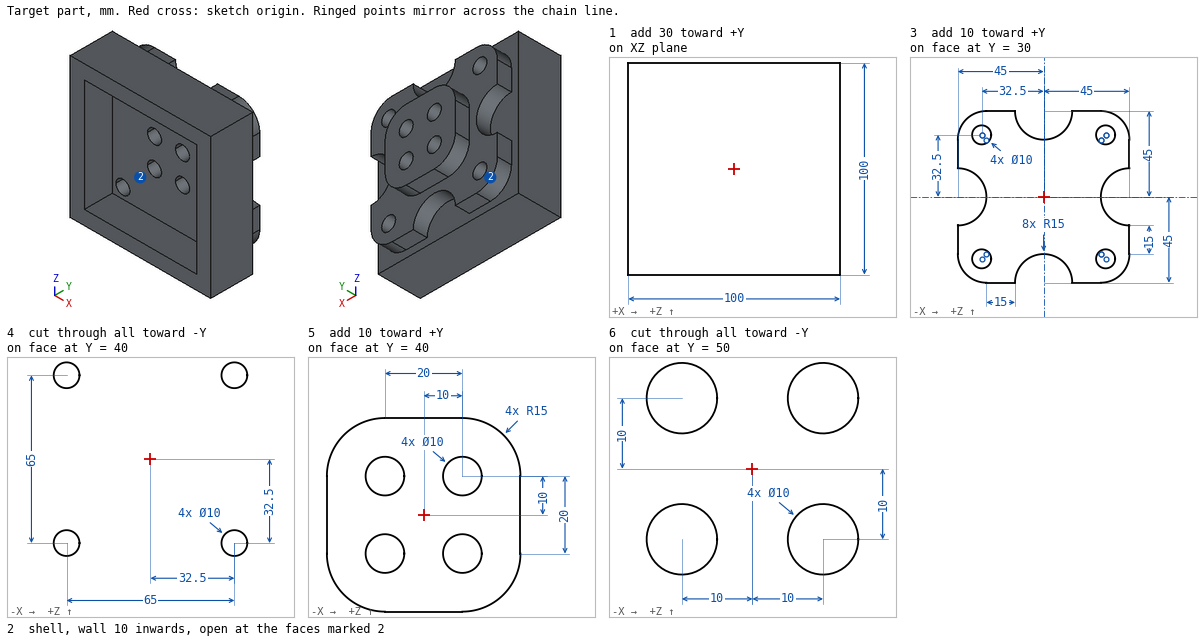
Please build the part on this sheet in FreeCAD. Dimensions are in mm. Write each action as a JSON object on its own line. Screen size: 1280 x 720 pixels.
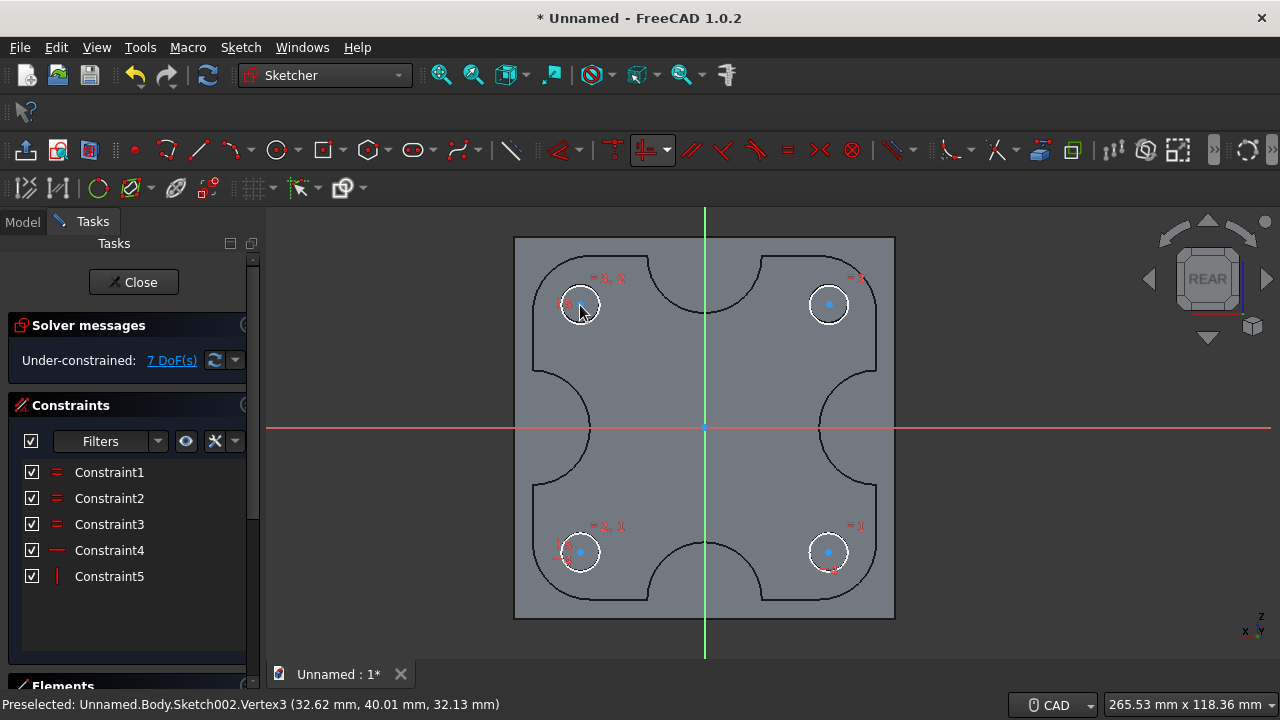
{"action": "left_click", "coordinate": [829, 553]}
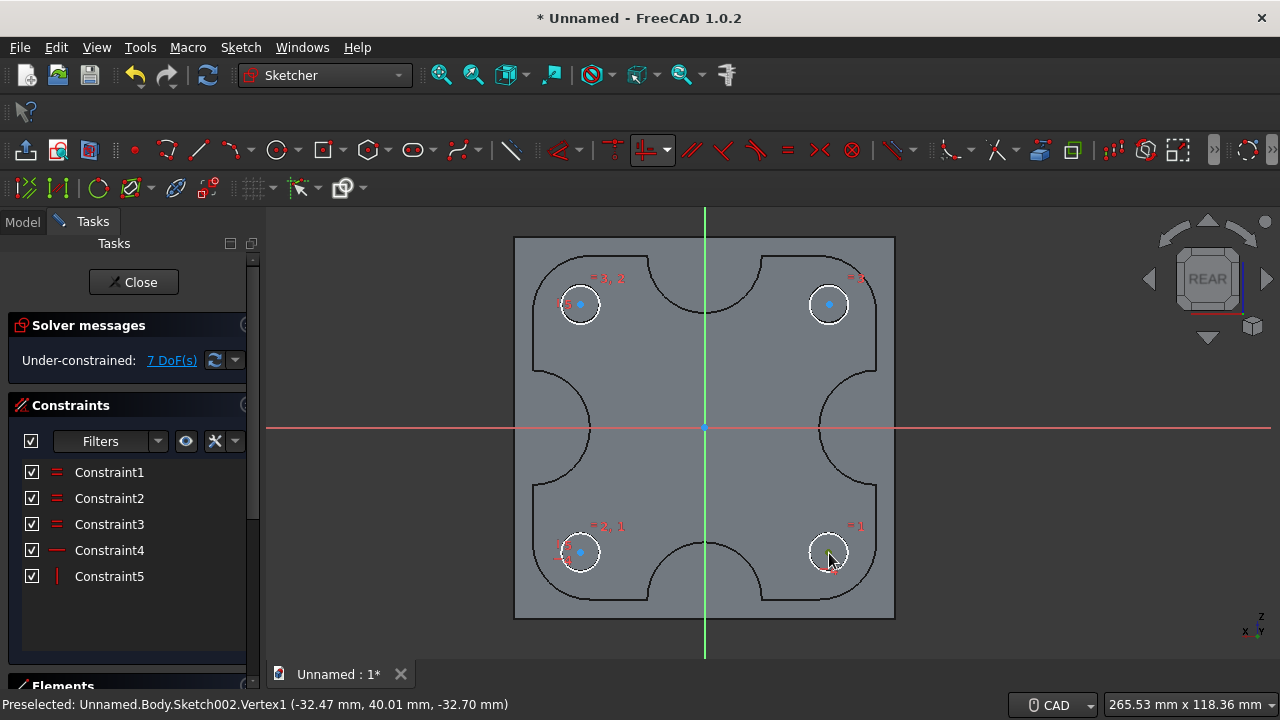
{"action": "left_click", "coordinate": [829, 305]}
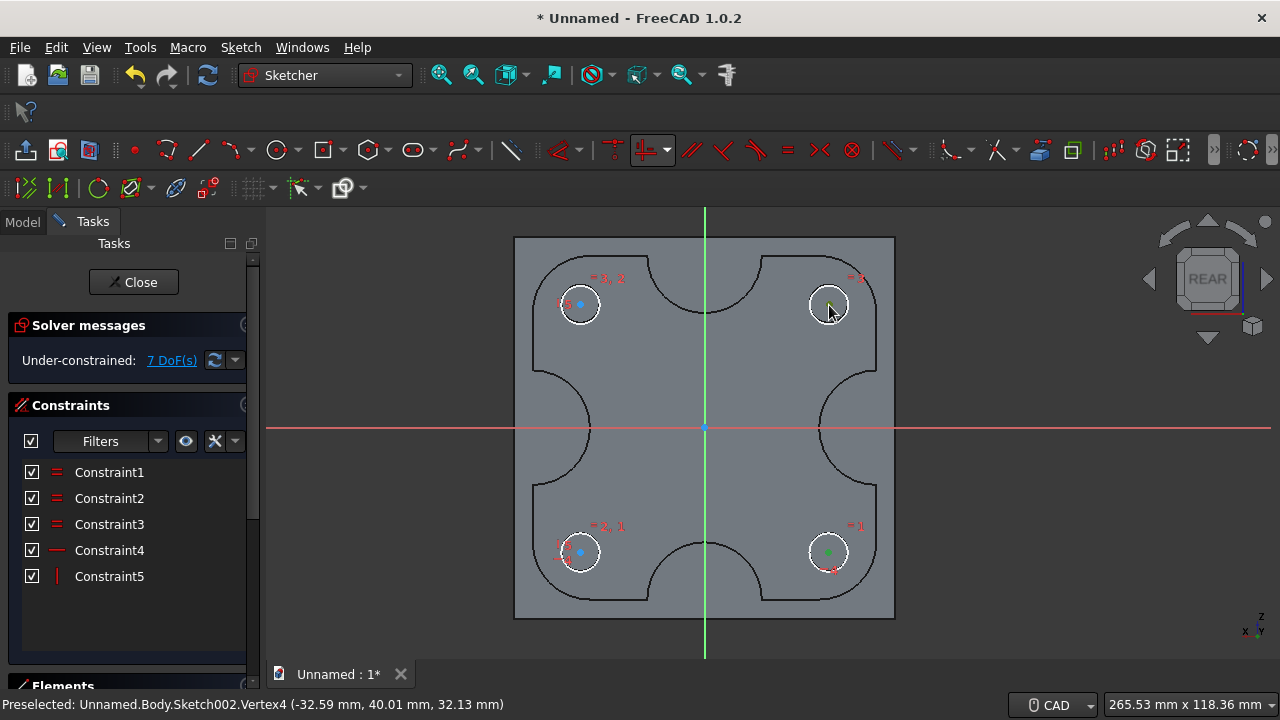
{"action": "key", "text": "v"}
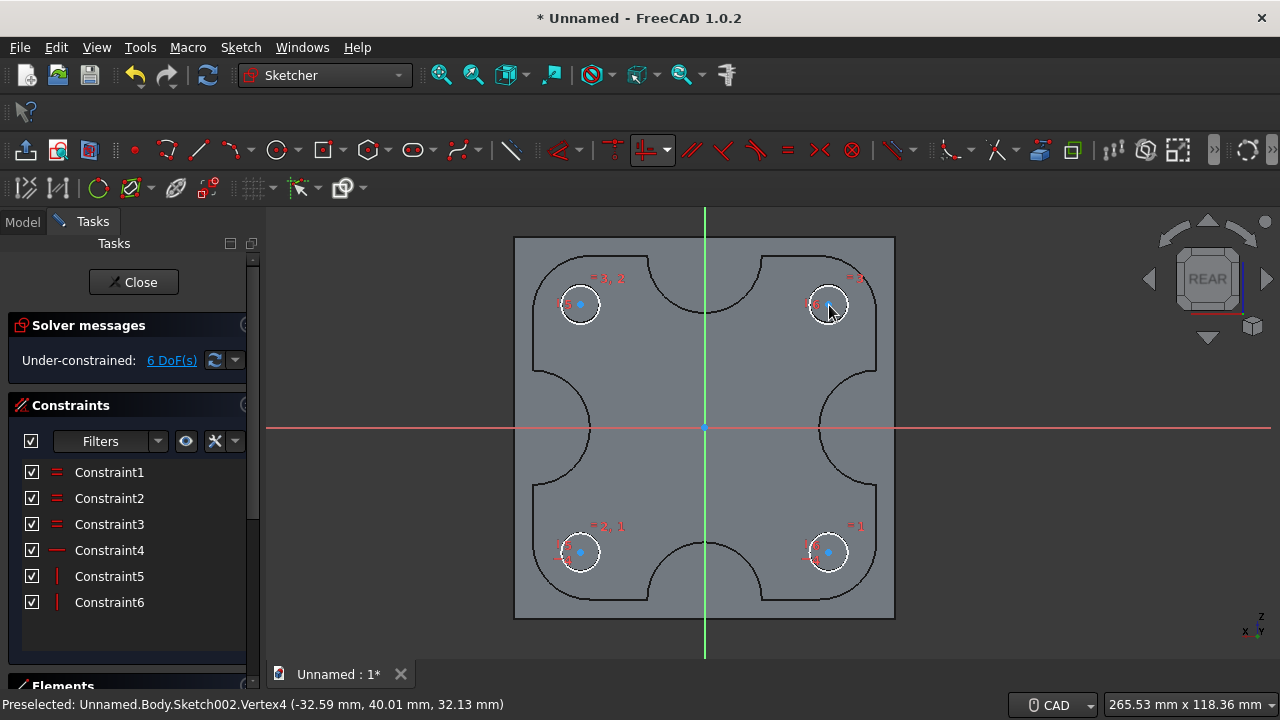
{"action": "left_click", "coordinate": [580, 305]}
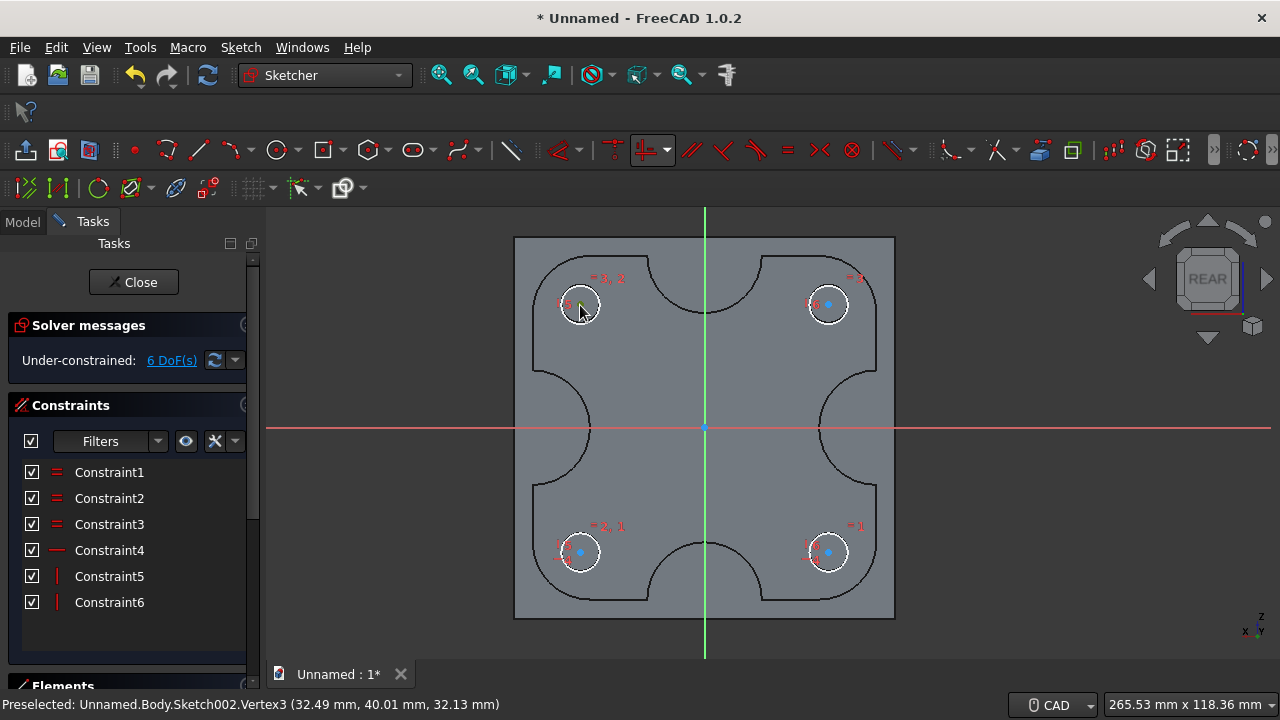
{"action": "left_click", "coordinate": [829, 305]}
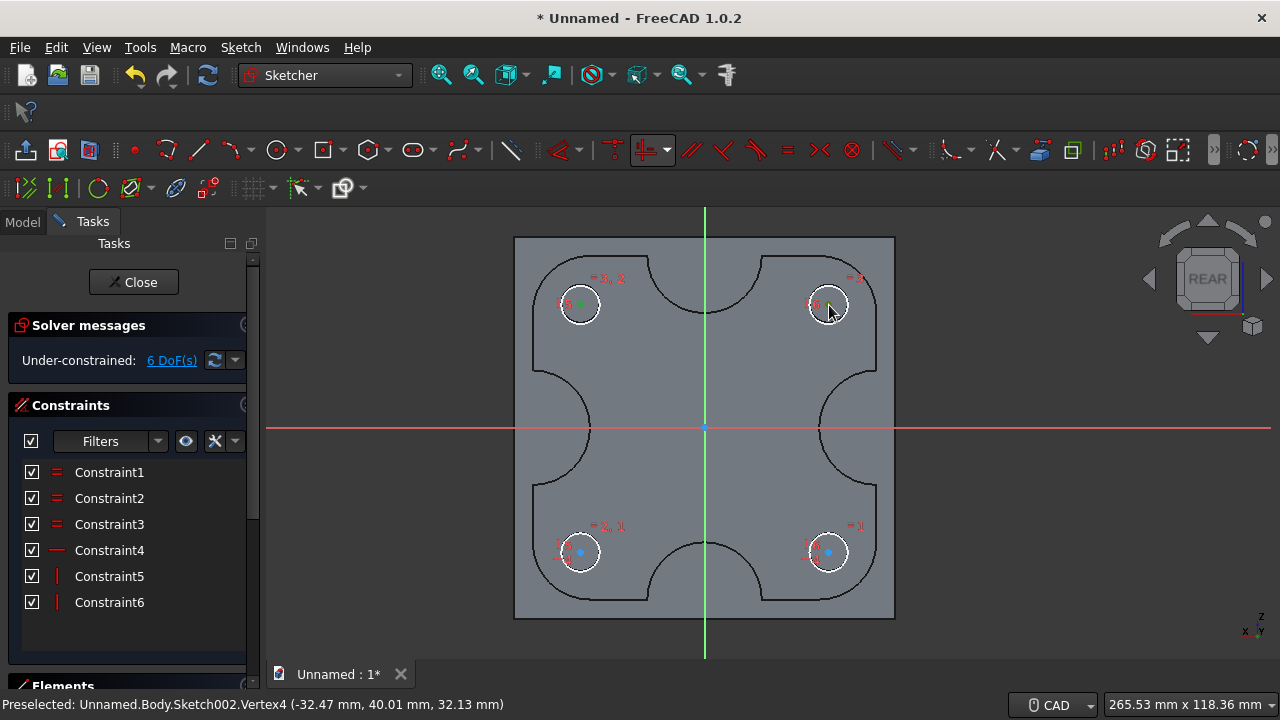
{"action": "key", "text": "h"}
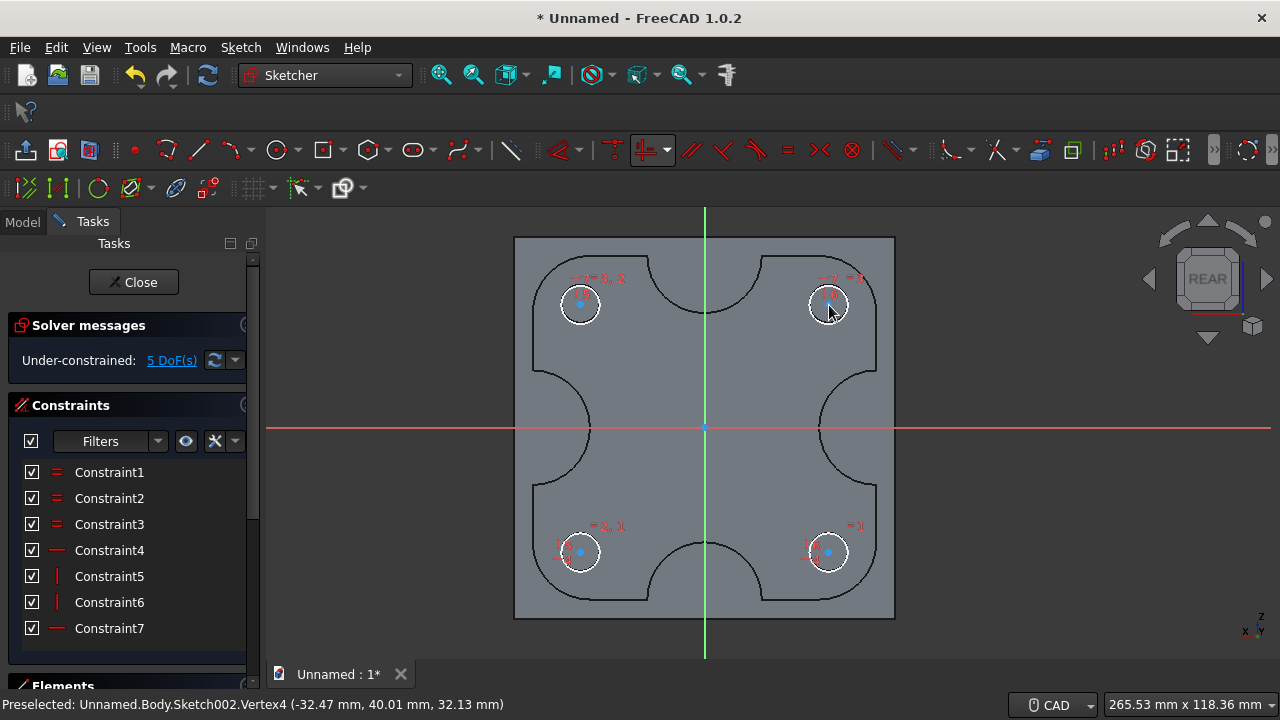
{"action": "left_click", "coordinate": [558, 150]}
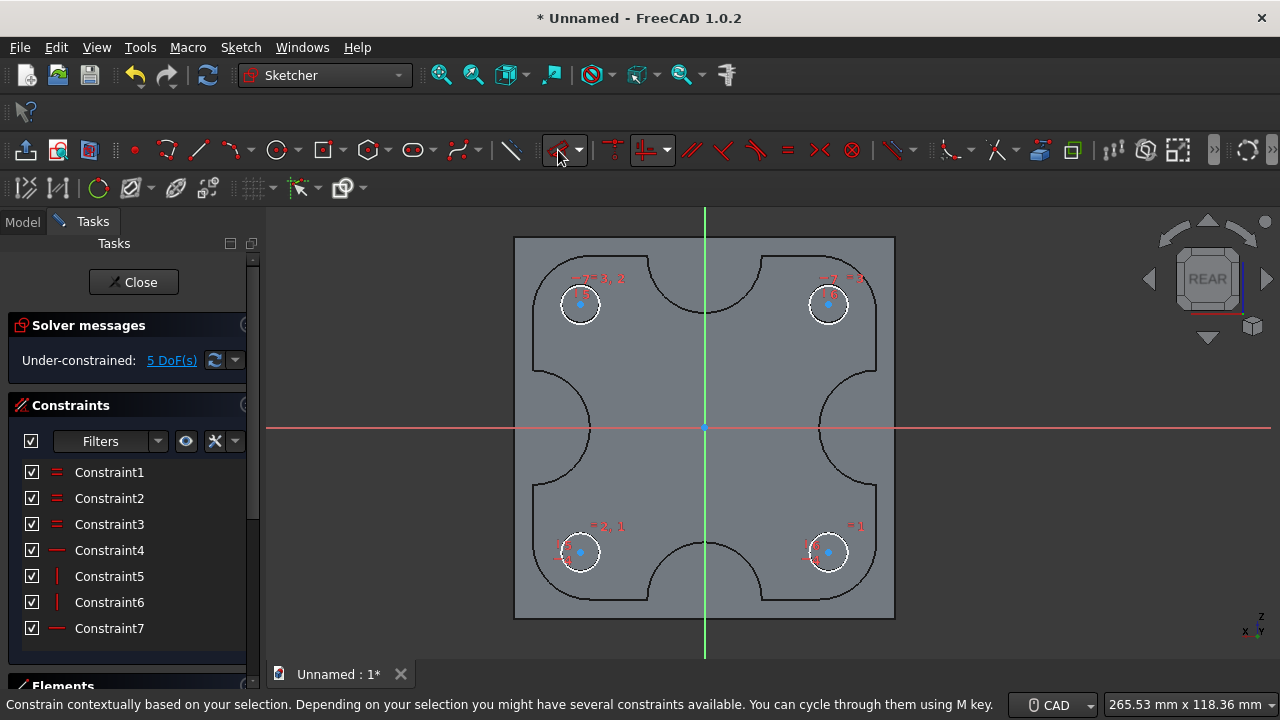
{"action": "left_click", "coordinate": [842, 539]}
{"action": "left_click", "coordinate": [865, 516]}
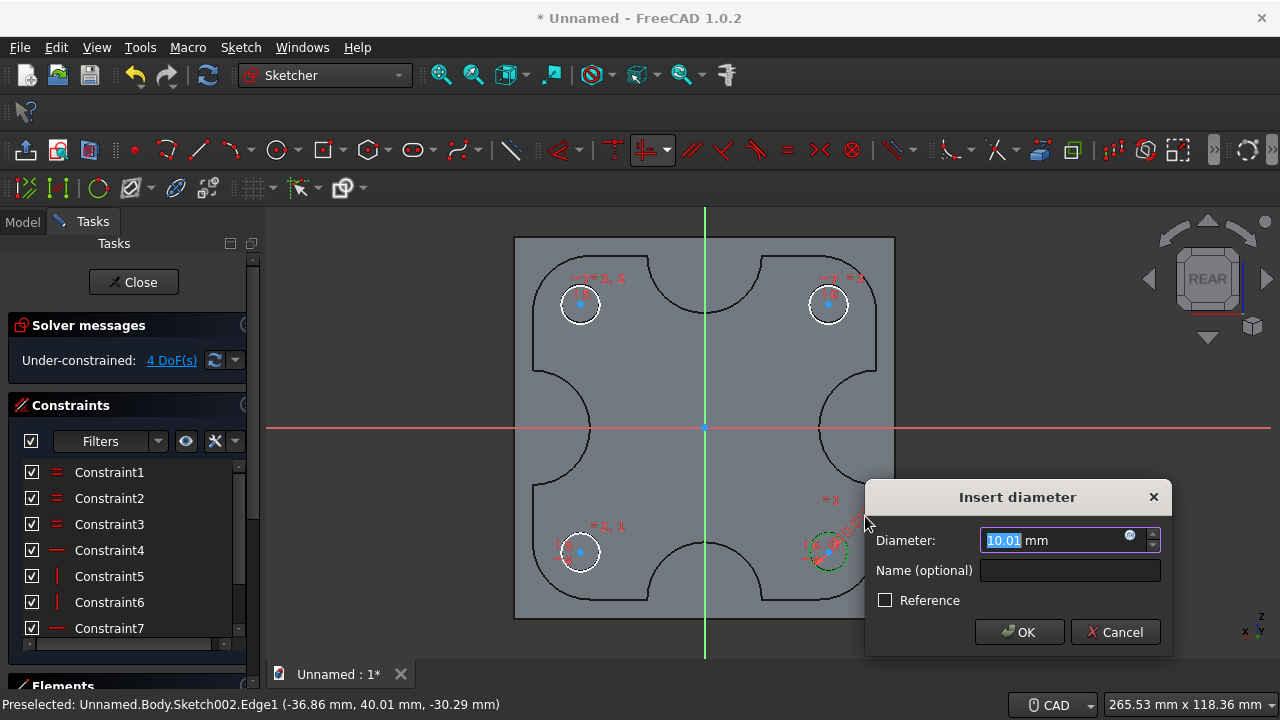
{"action": "type", "text": "10"}
{"action": "key", "text": "Return"}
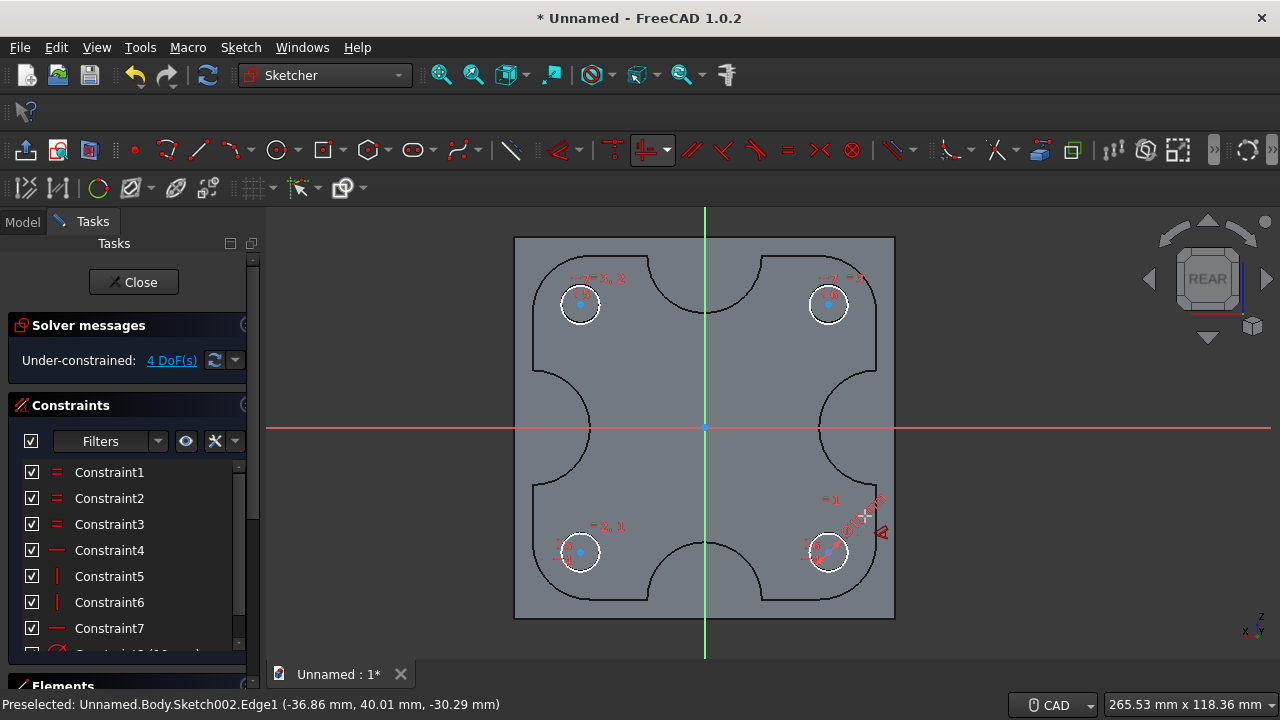
{"action": "left_click", "coordinate": [829, 553]}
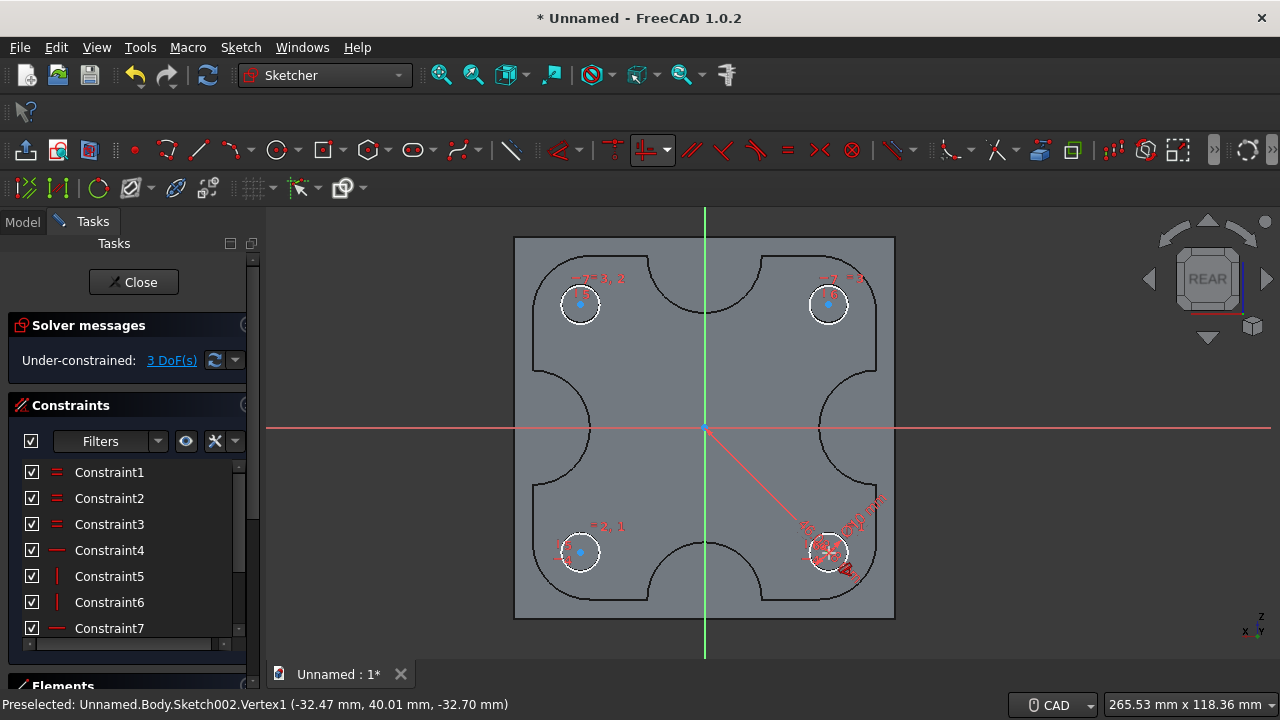
{"action": "left_click", "coordinate": [580, 553]}
{"action": "left_click", "coordinate": [647, 587]}